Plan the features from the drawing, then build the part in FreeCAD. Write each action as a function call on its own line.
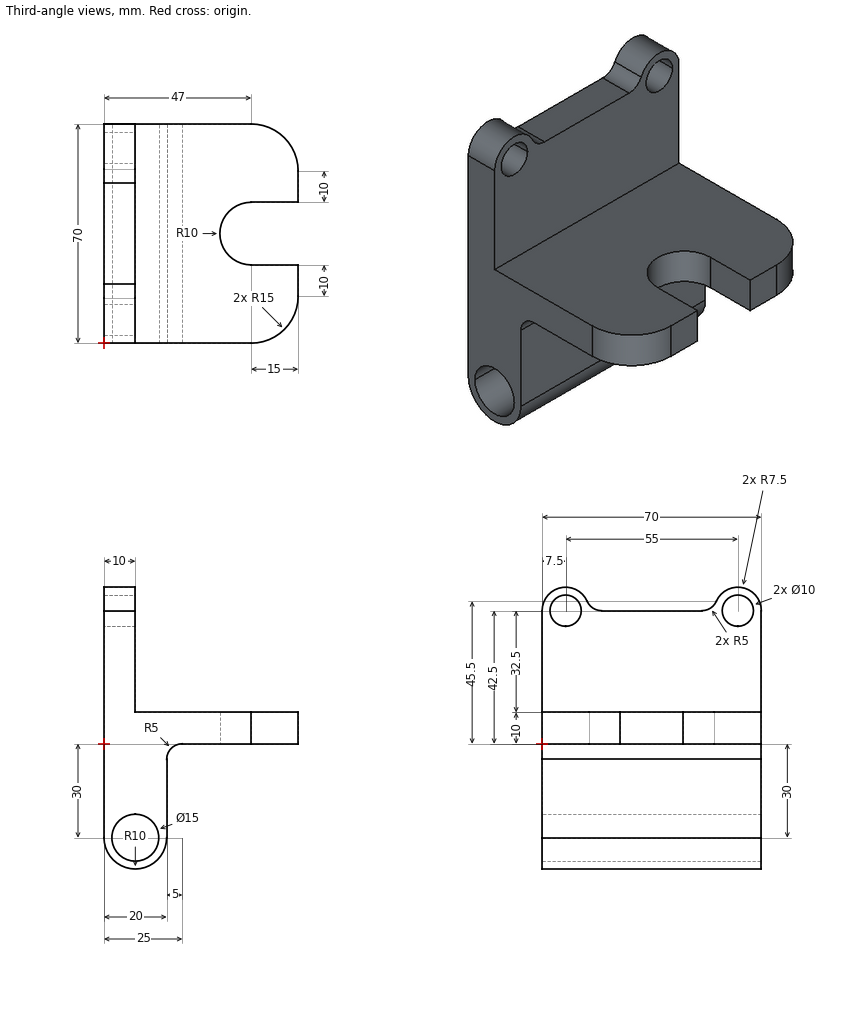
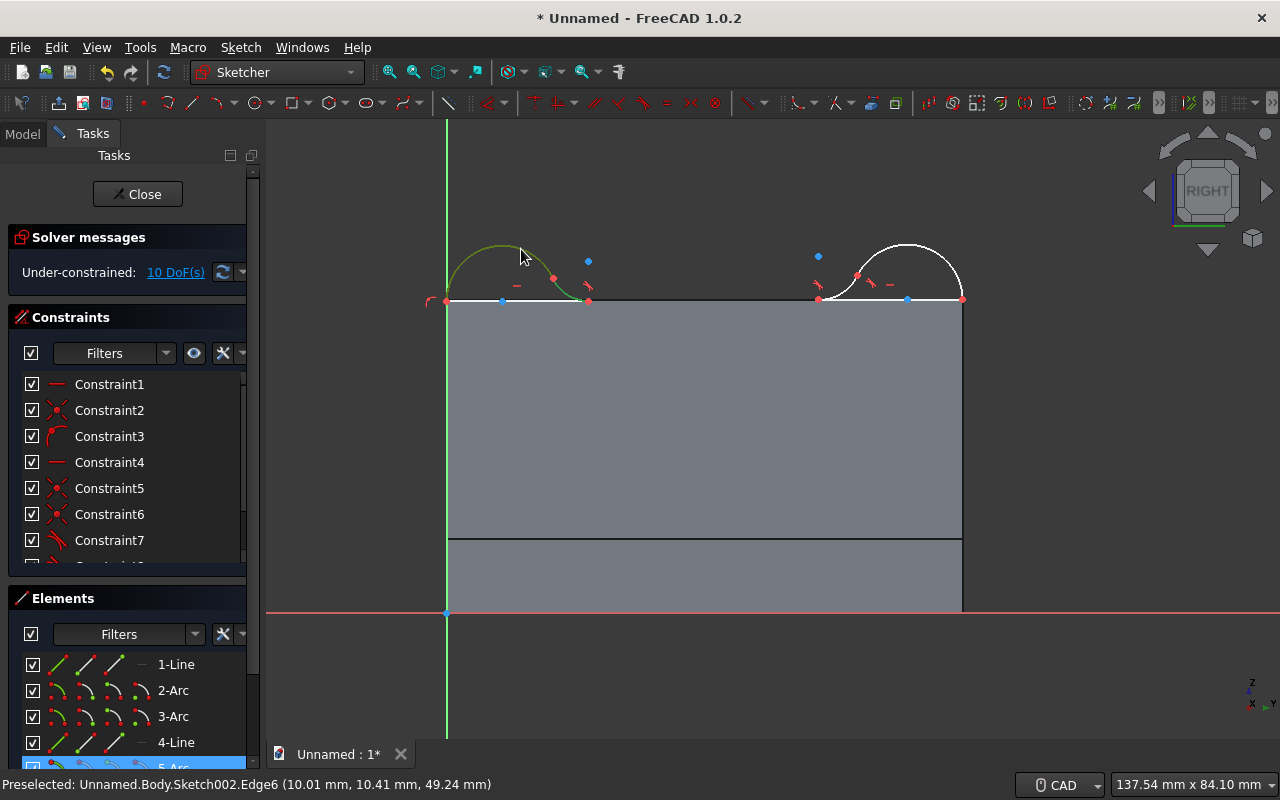
click(644, 104)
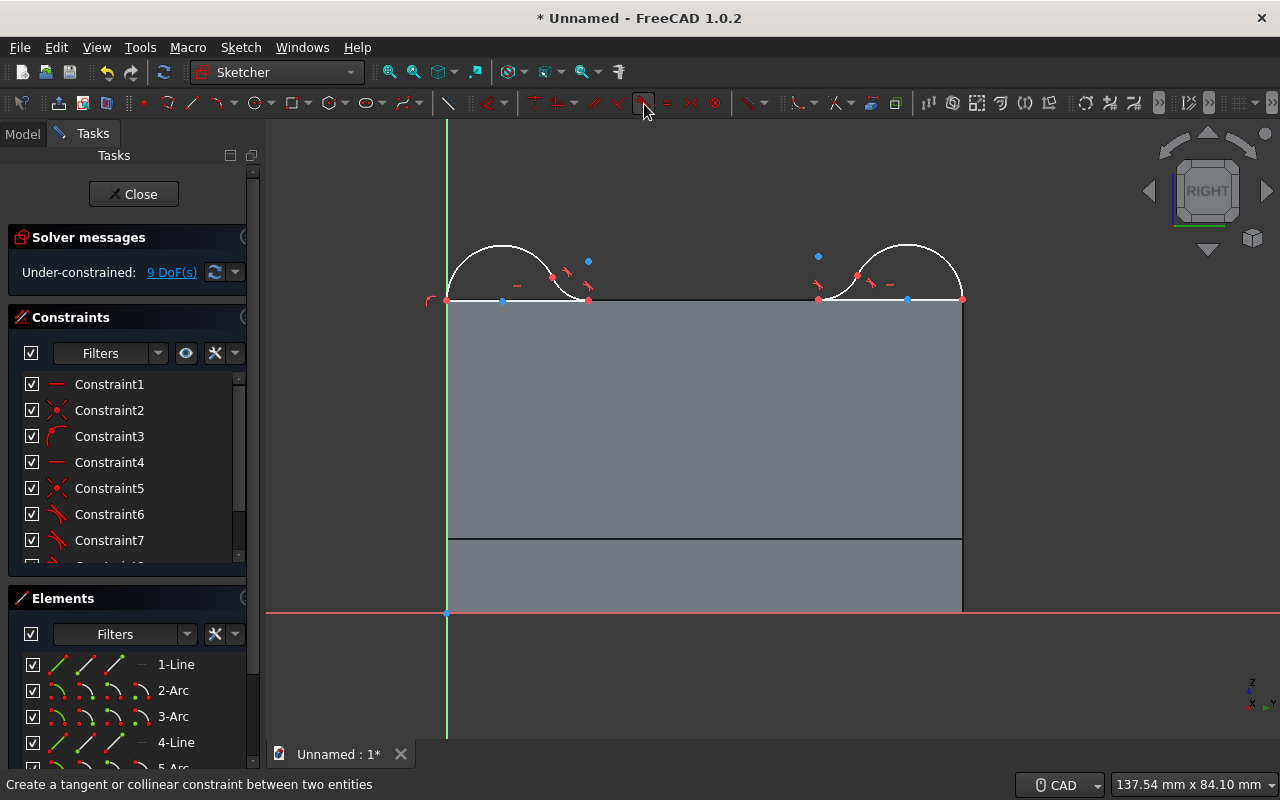
click(849, 287)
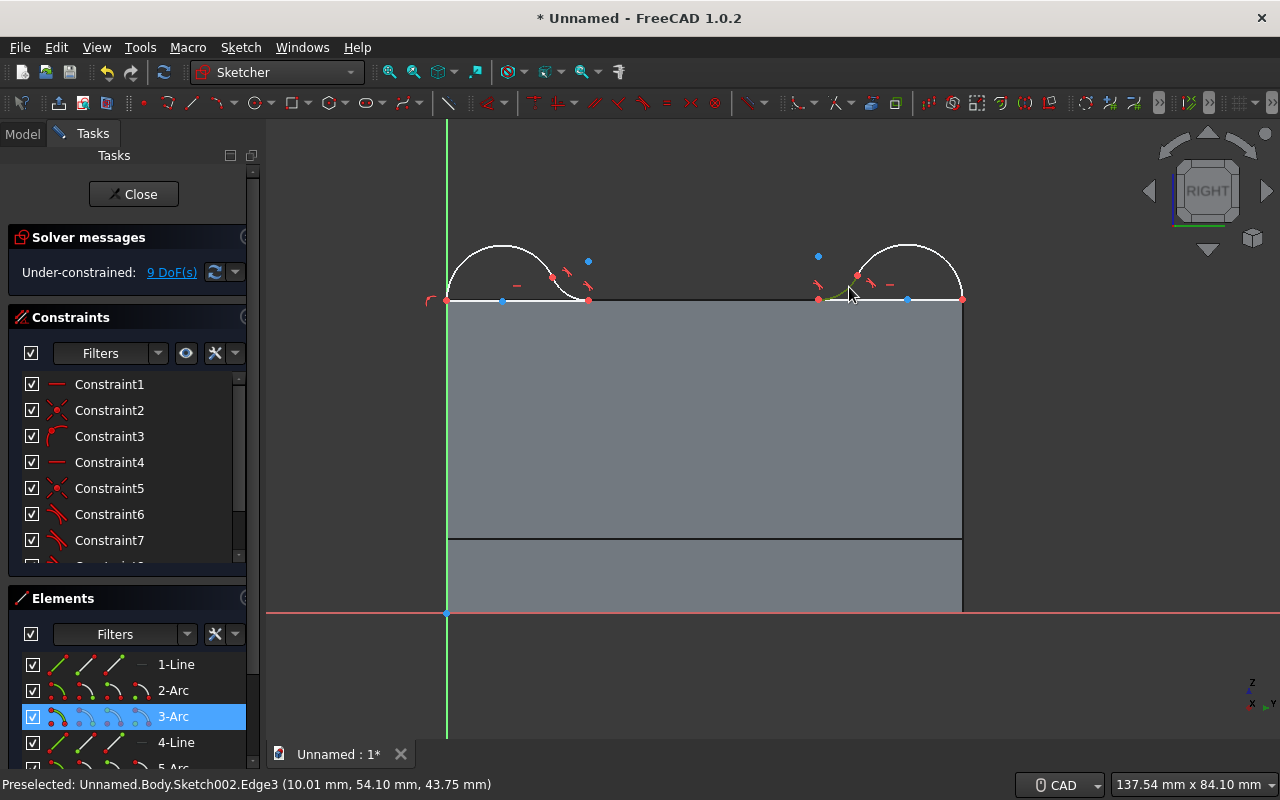
click(561, 289)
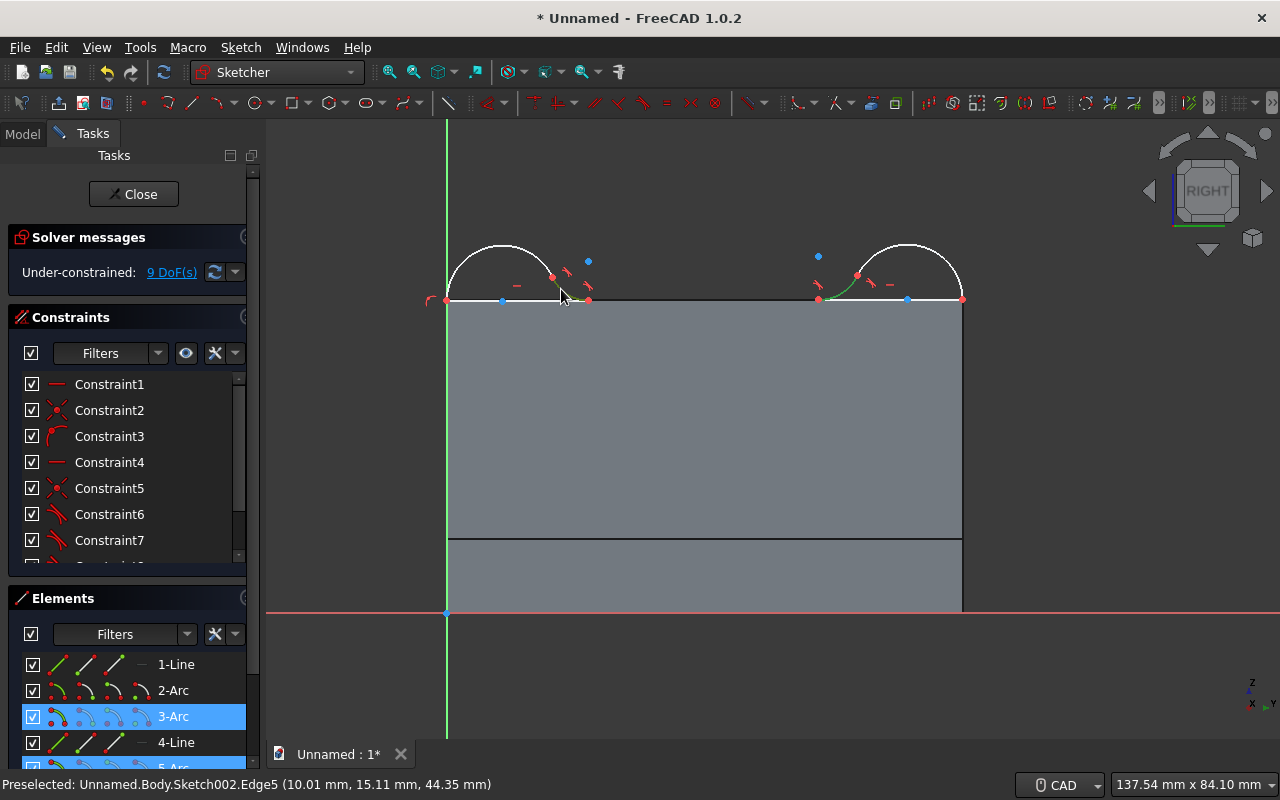
click(668, 104)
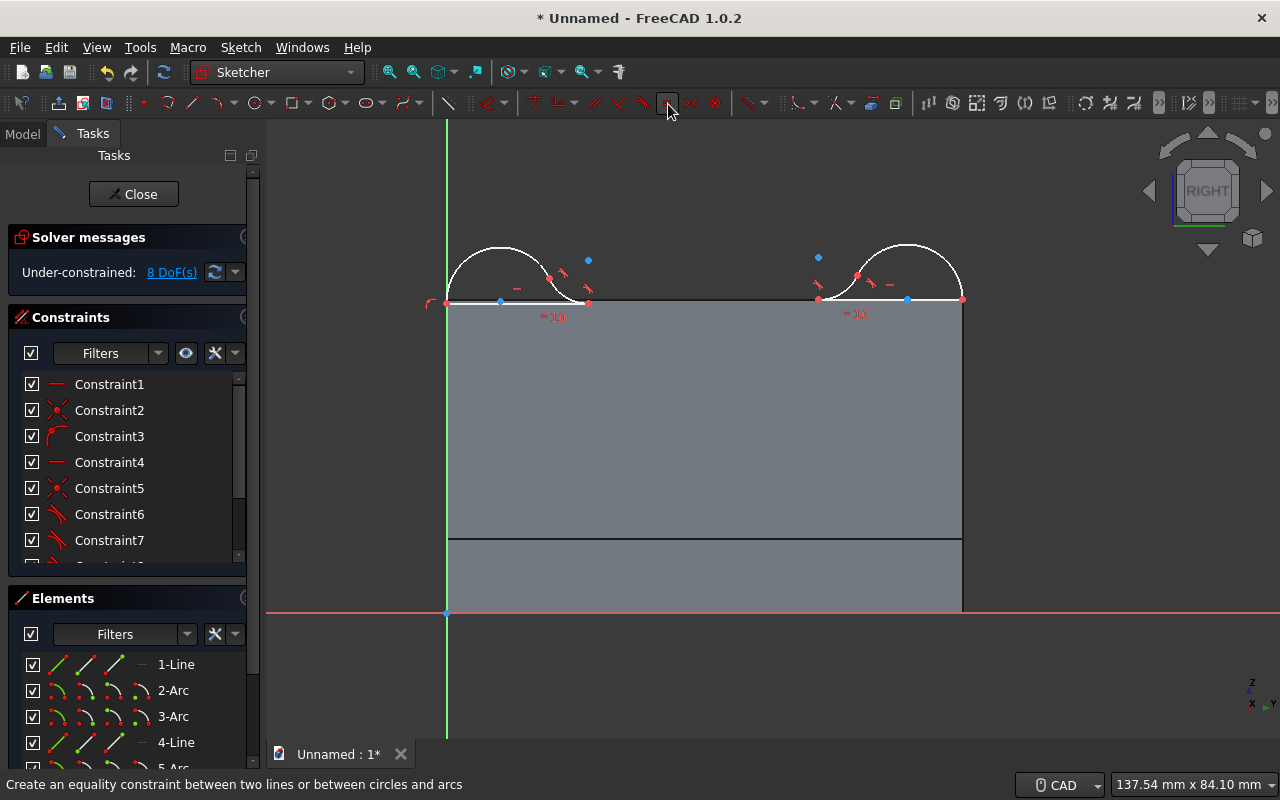
click(945, 260)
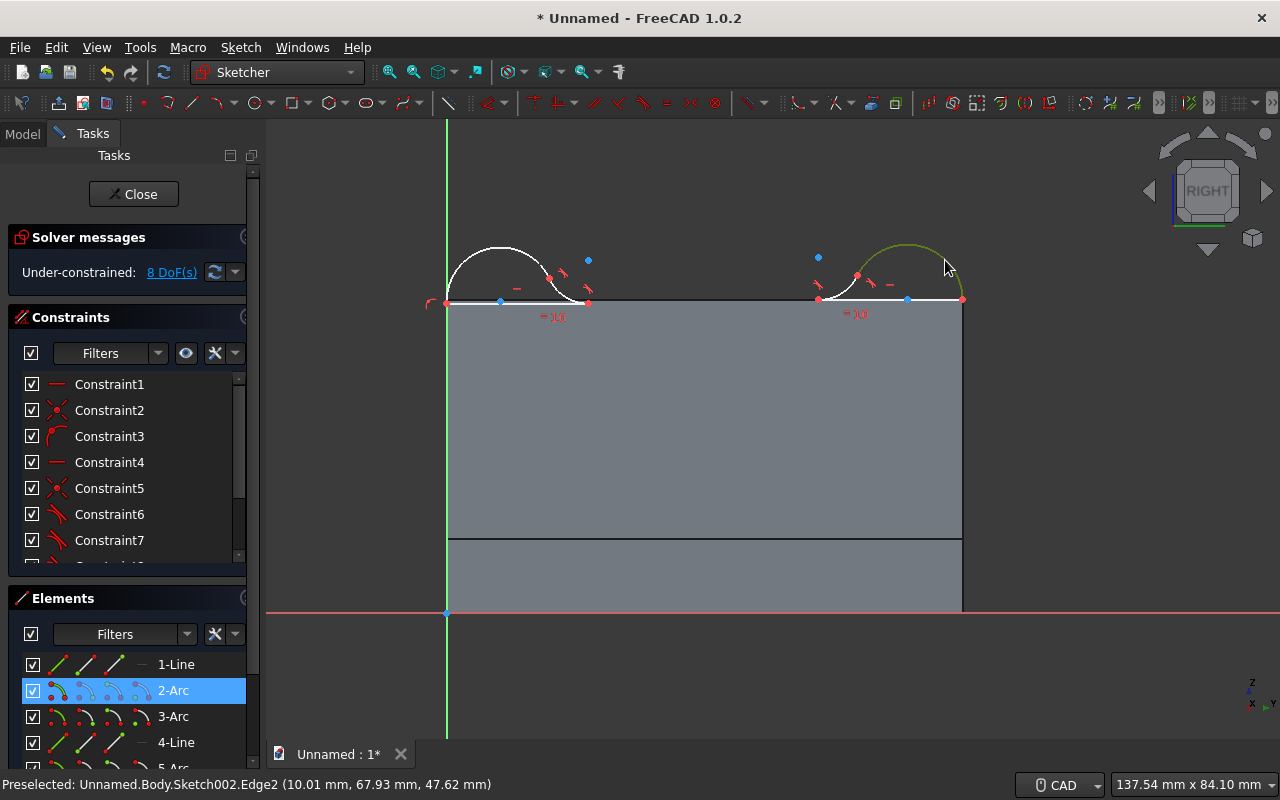
click(517, 250)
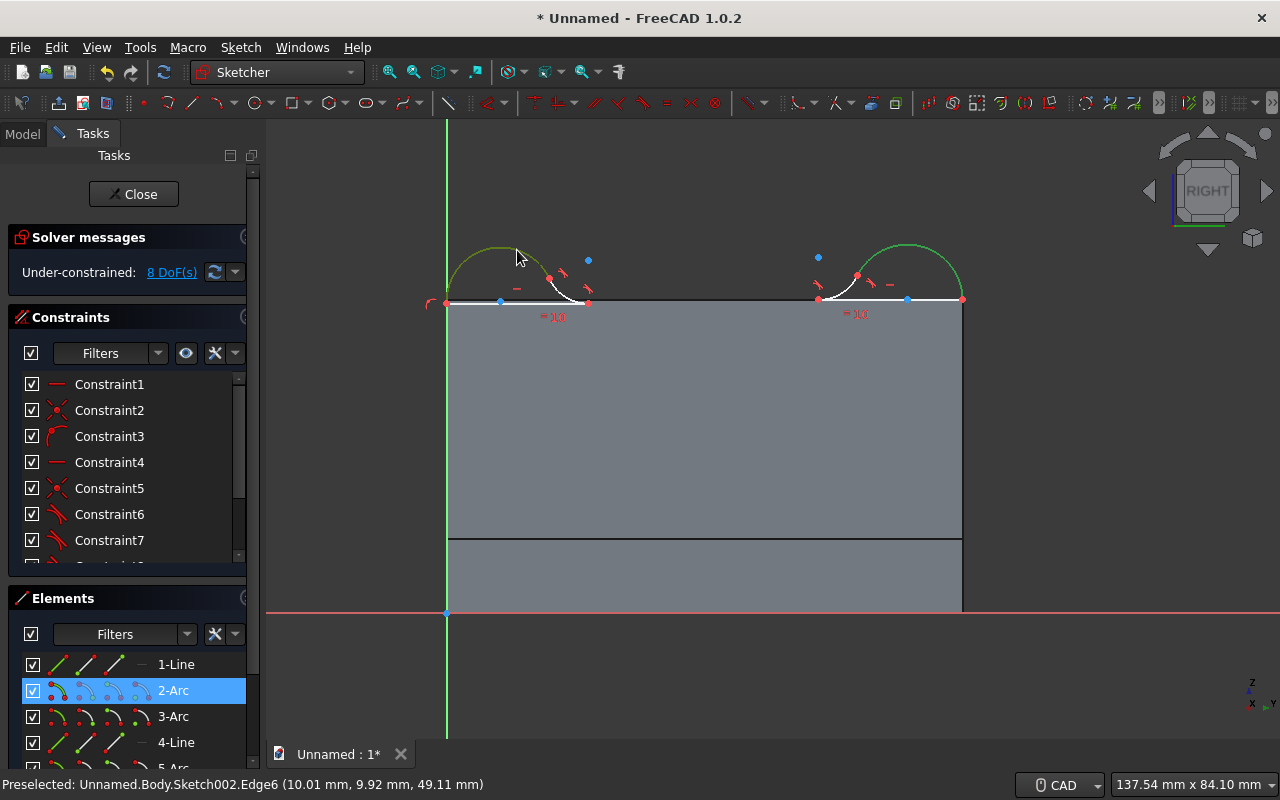
click(668, 104)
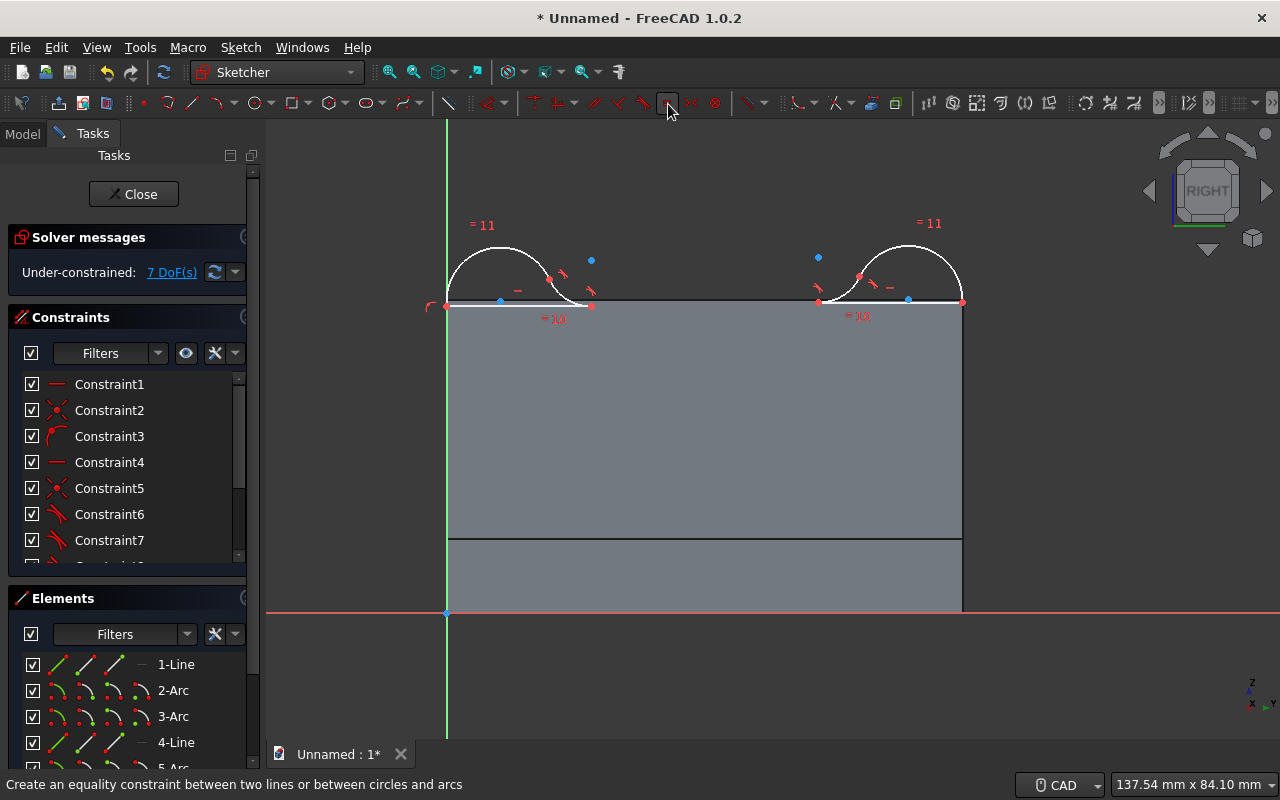
click(488, 104)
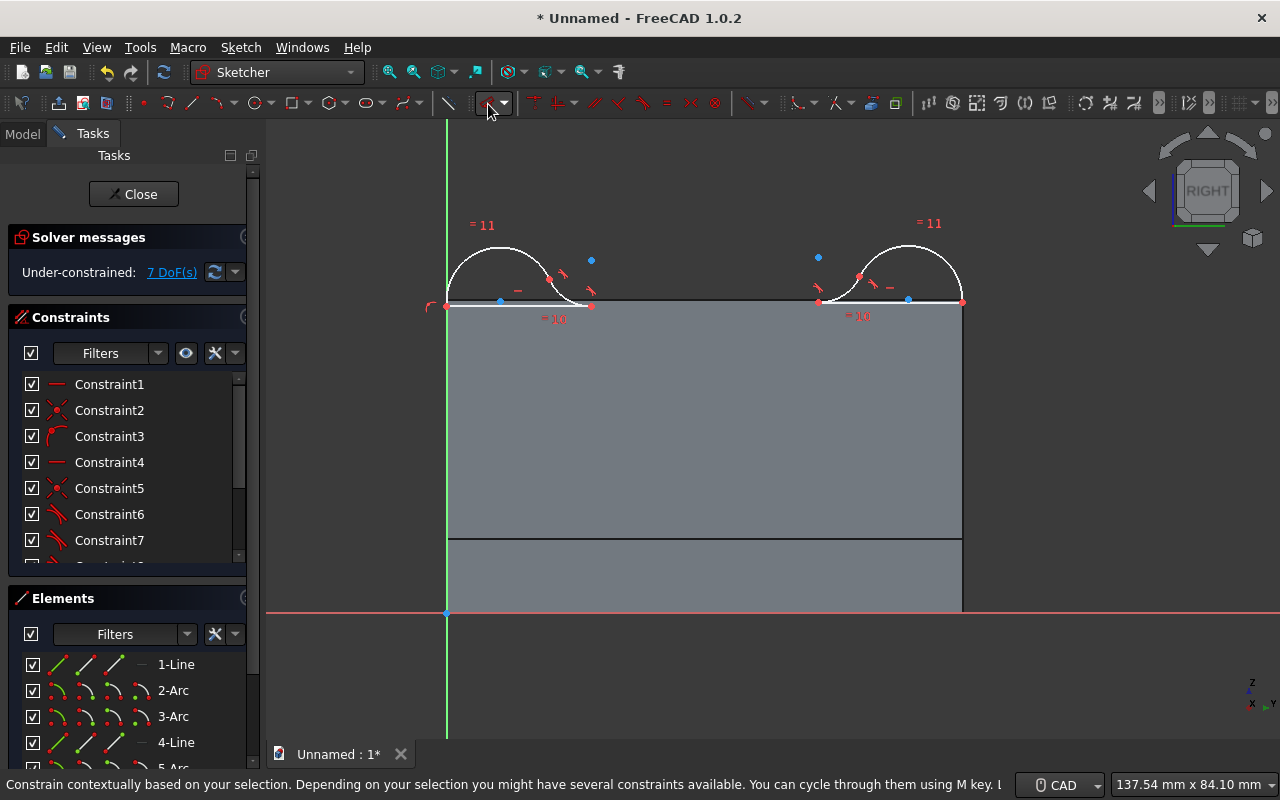
click(947, 262)
click(970, 240)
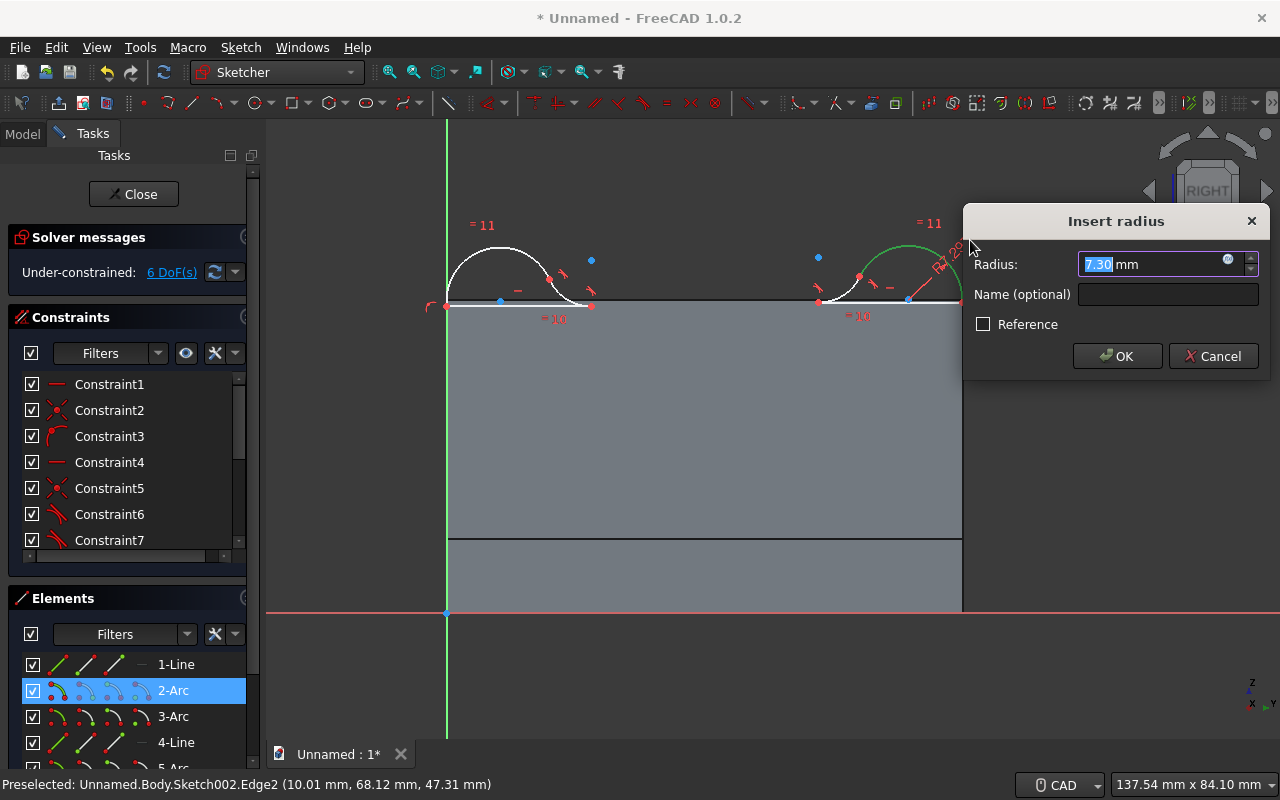
text(7.5)
key(Return)